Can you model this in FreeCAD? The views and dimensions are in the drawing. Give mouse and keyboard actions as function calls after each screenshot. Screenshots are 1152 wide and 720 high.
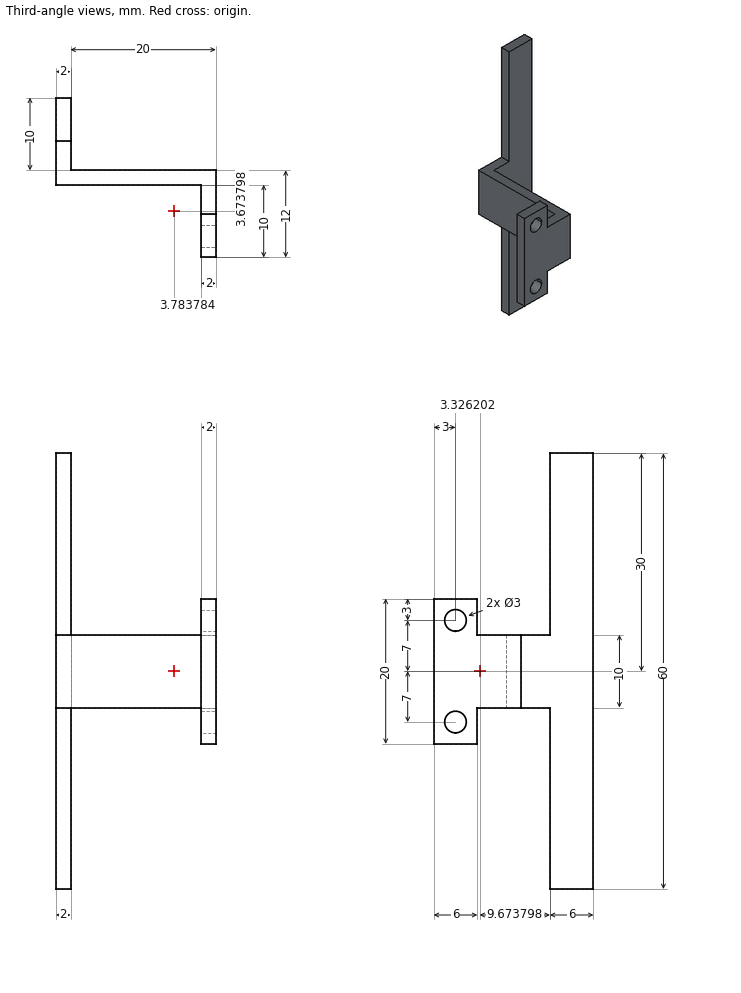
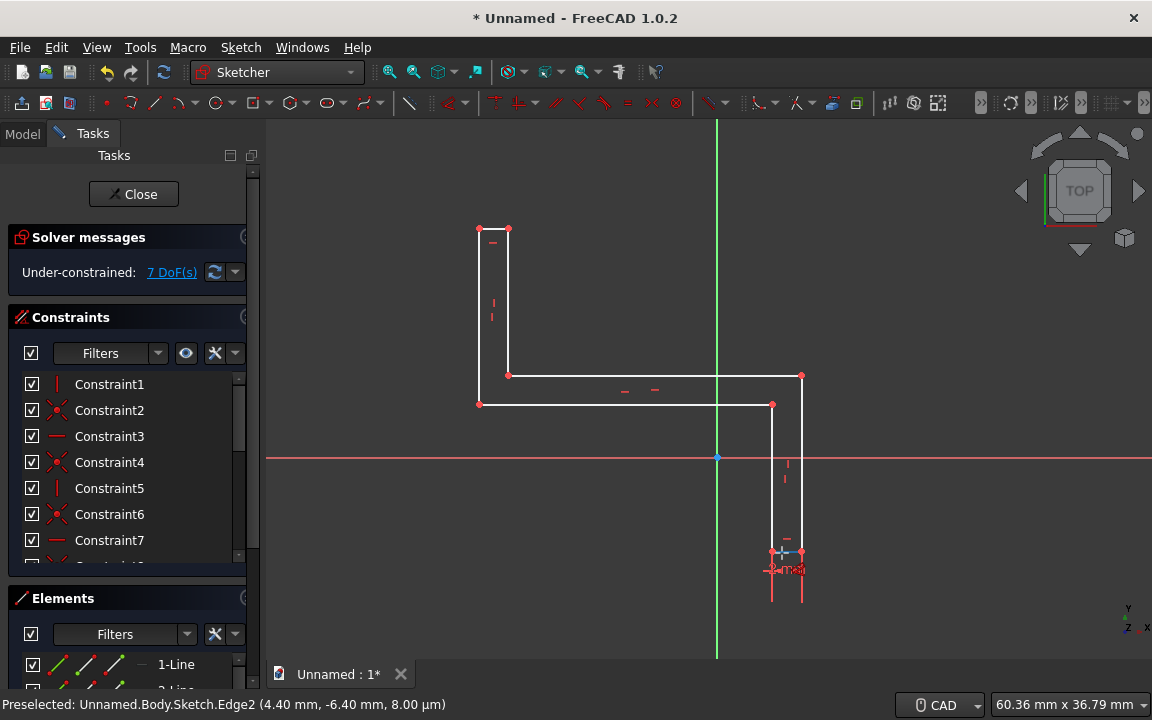
scroll(500, 229, up, 3)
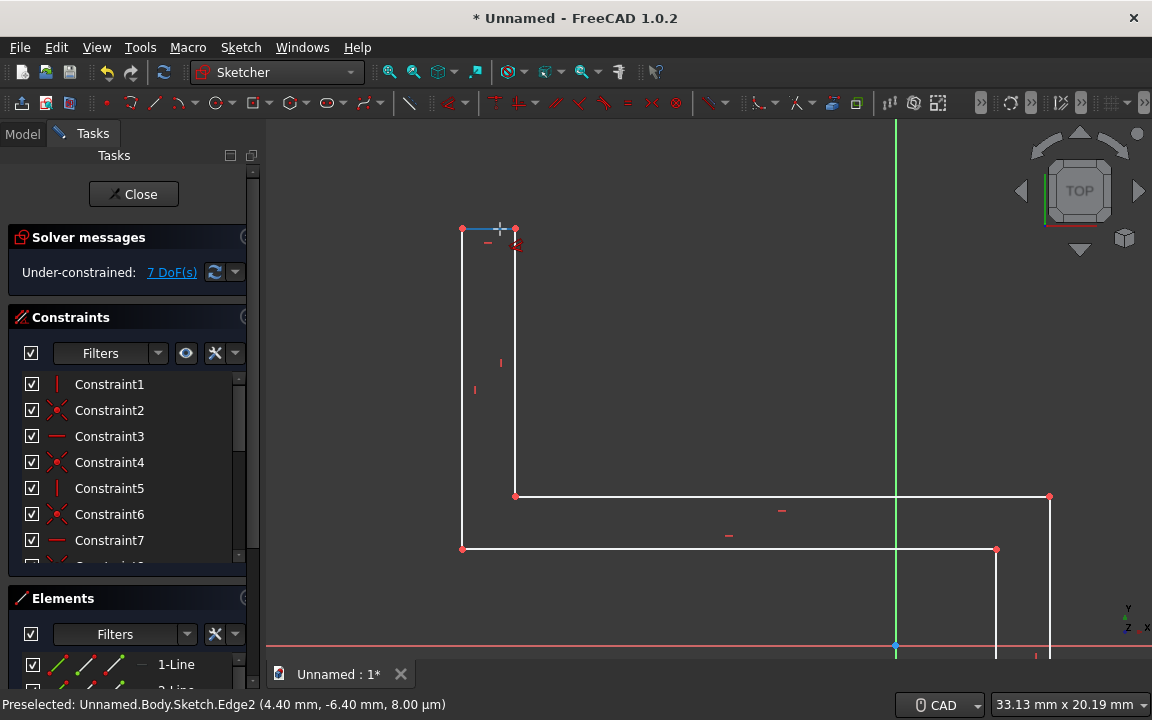
click(499, 229)
click(489, 195)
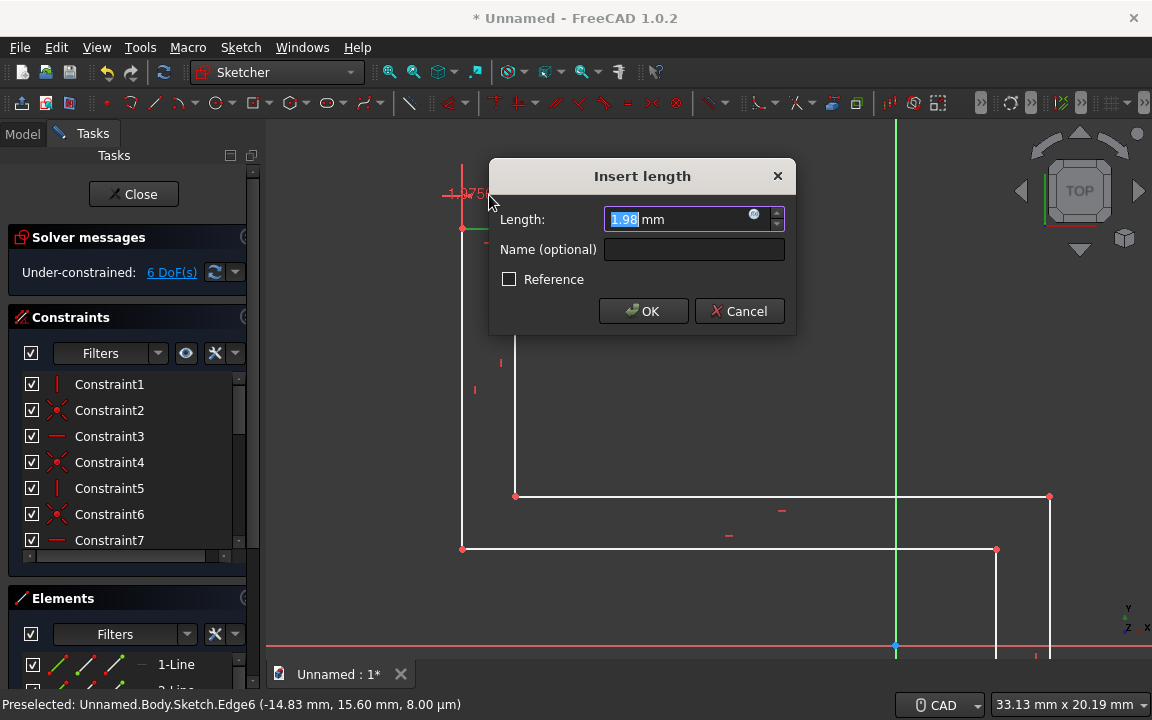
text(2)
key(Return)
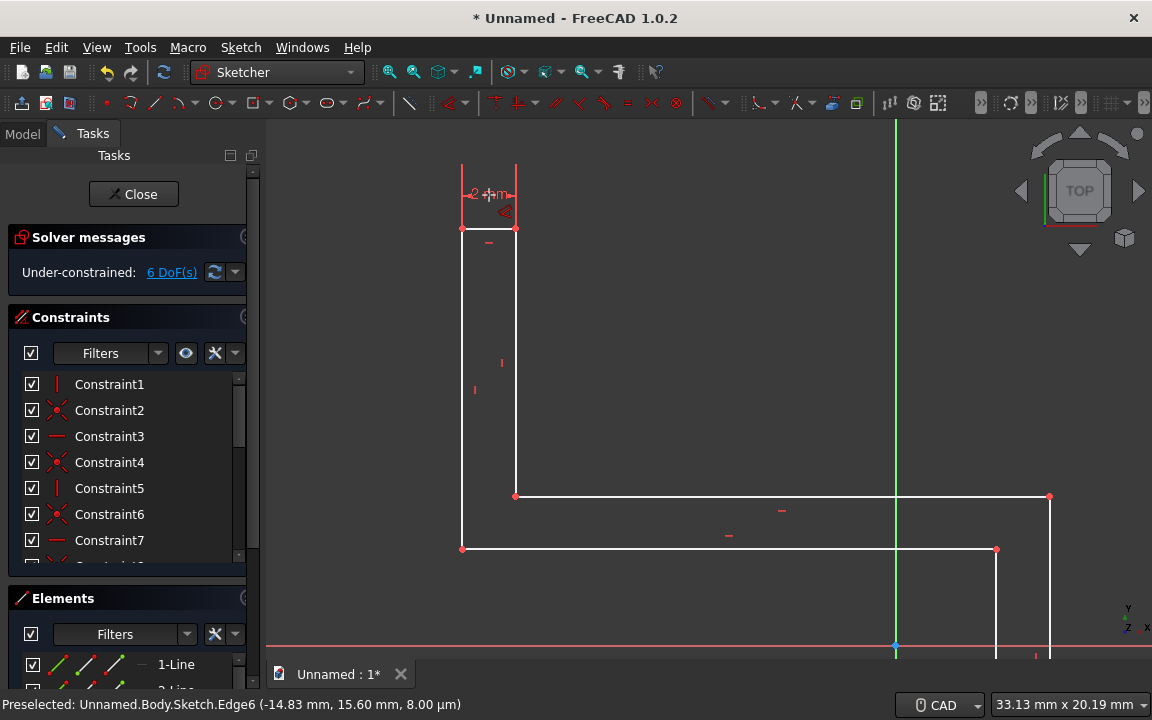
scroll(500, 229, down, 3)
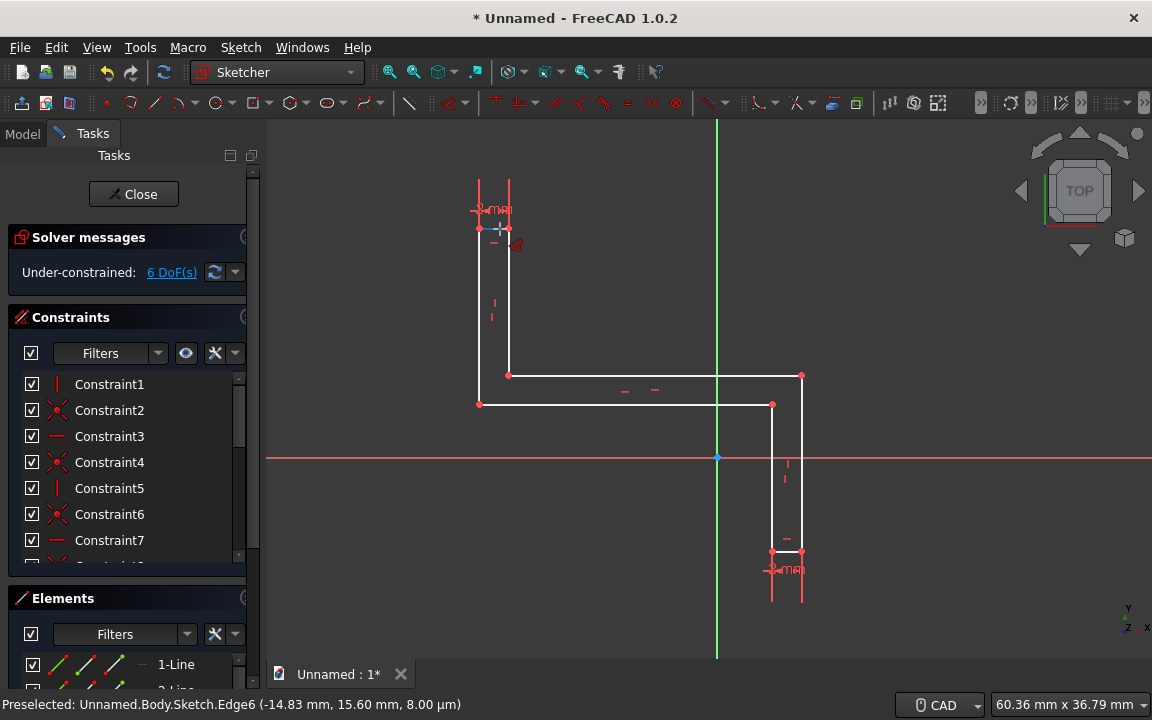
scroll(772, 449, up, 3)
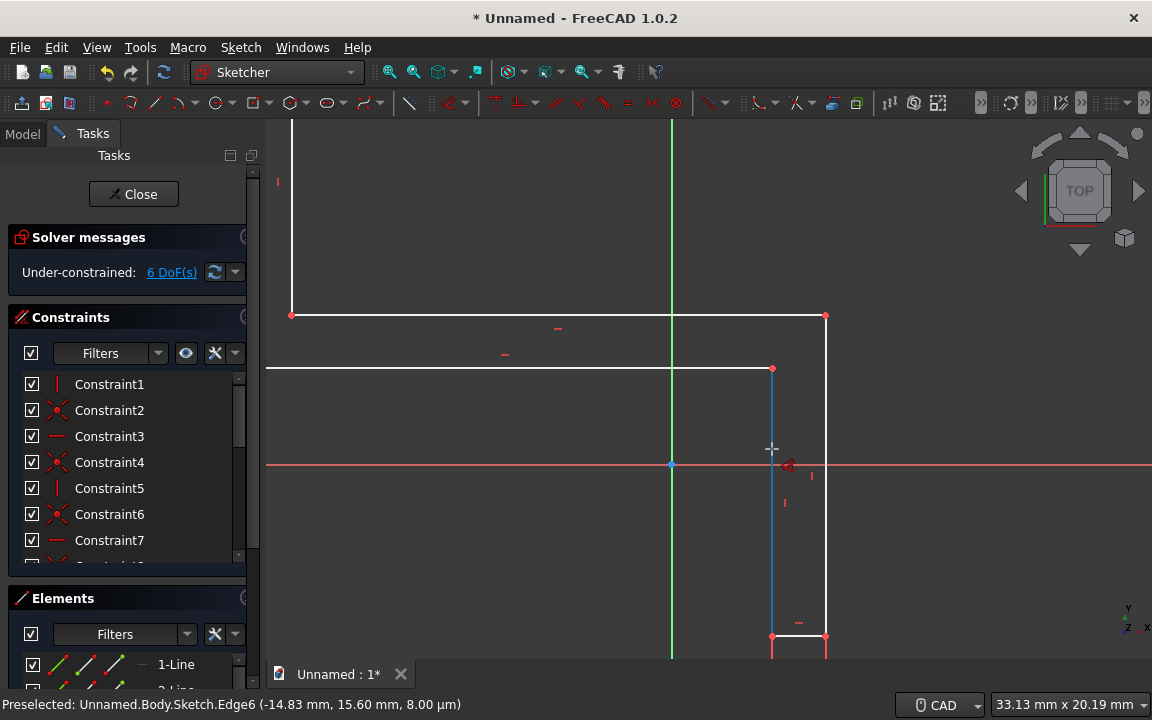
click(772, 449)
click(806, 500)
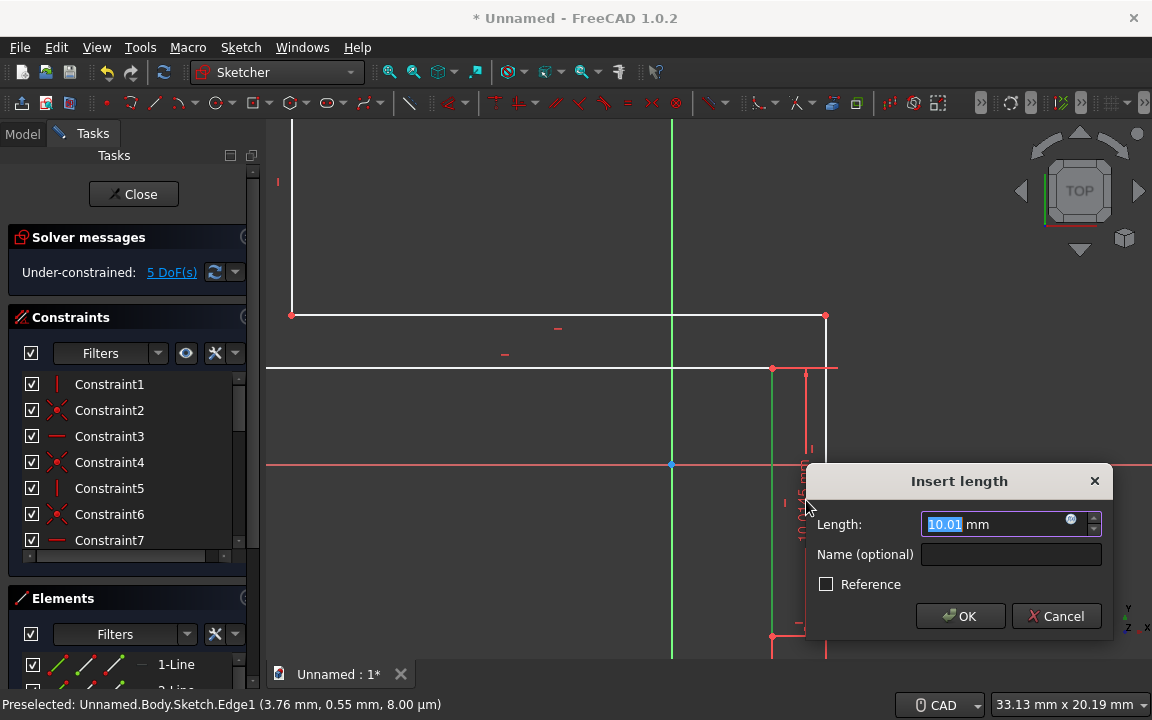
text(10)
key(Return)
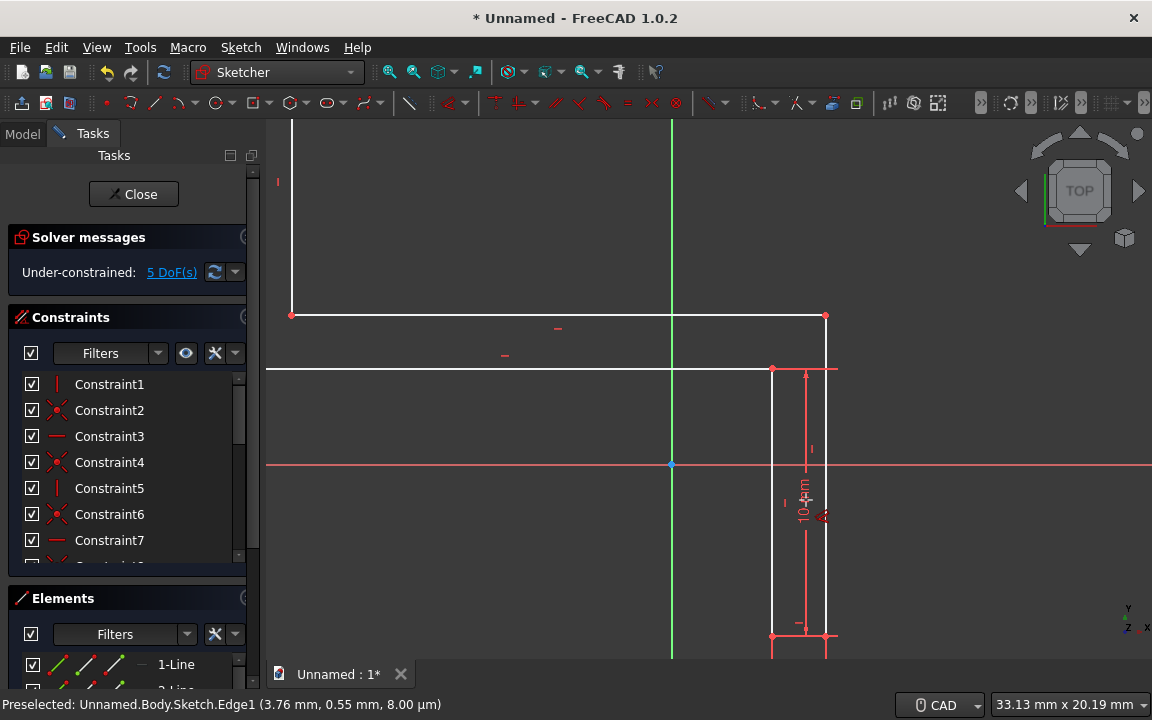
click(826, 540)
click(860, 401)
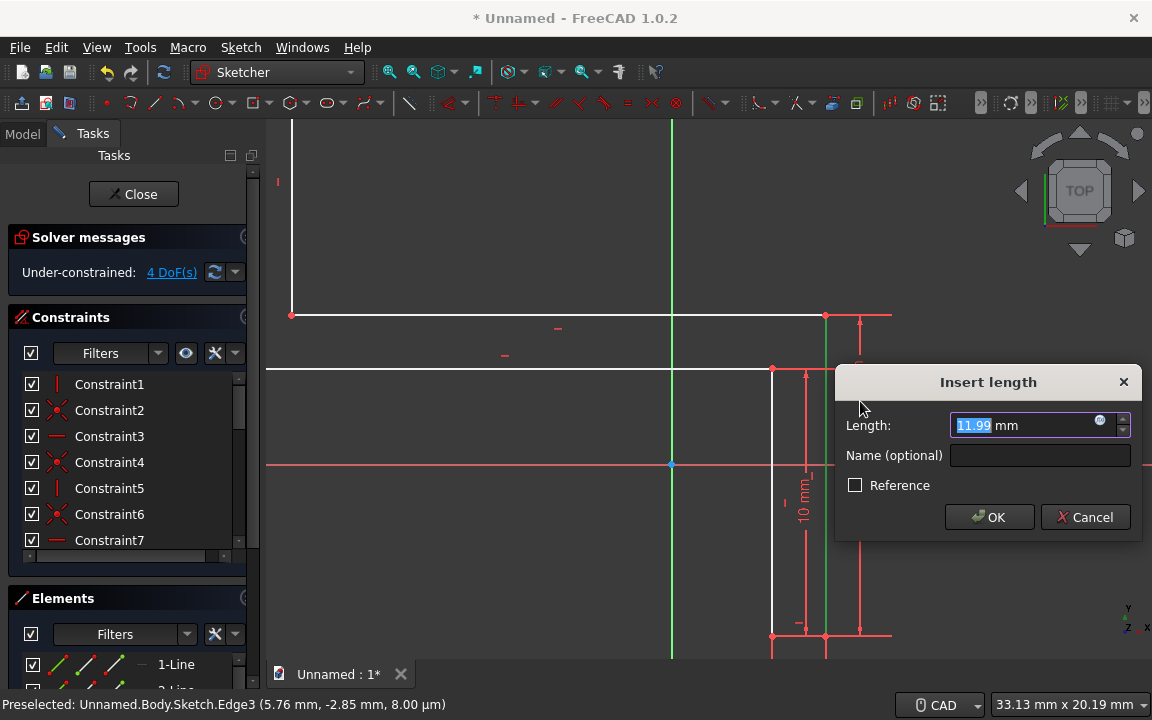
text(12)
key(Return)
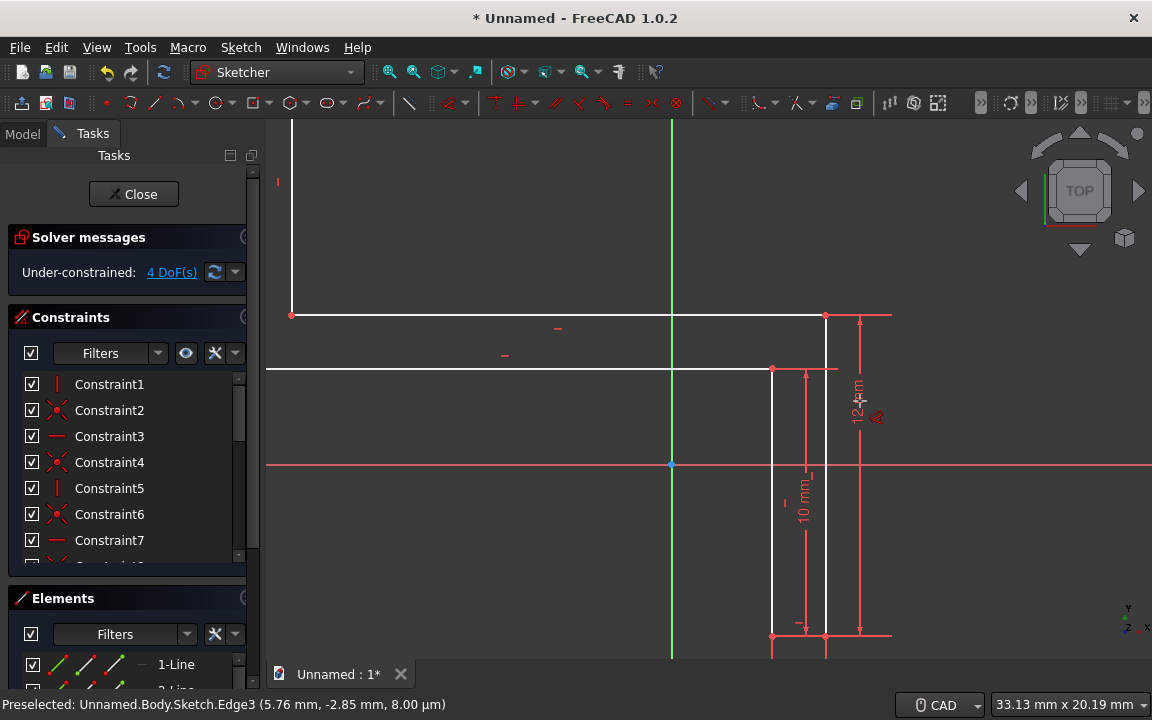
click(452, 315)
click(560, 281)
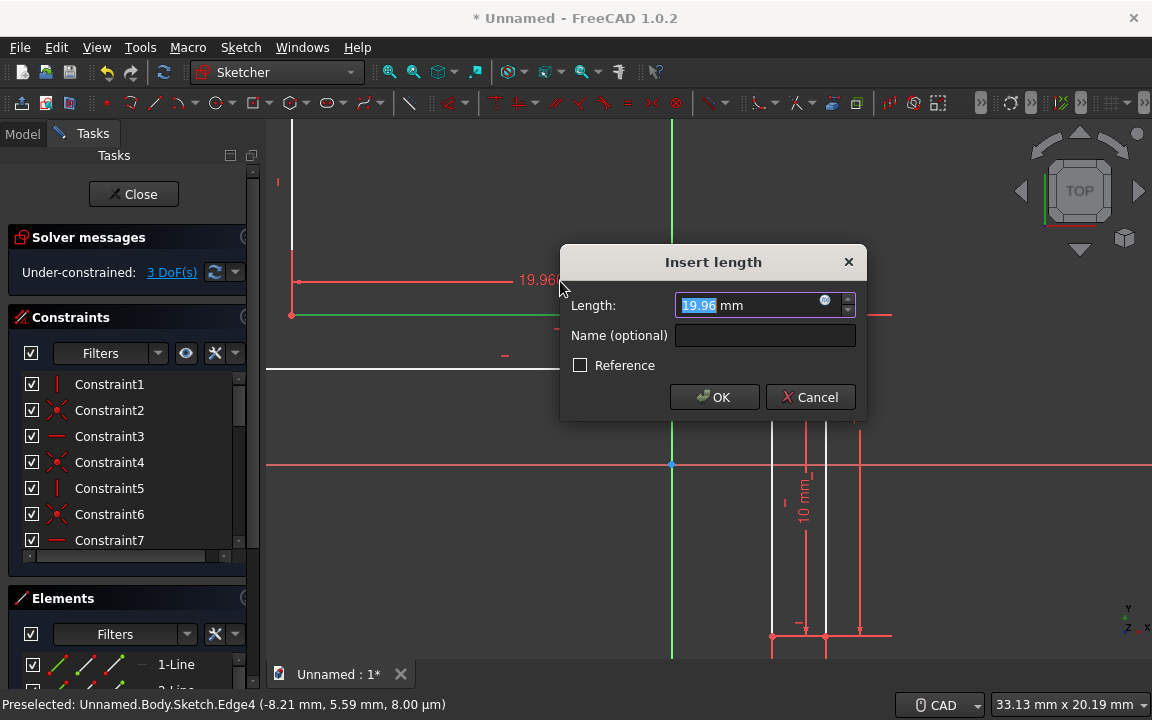
text(20)
key(Return)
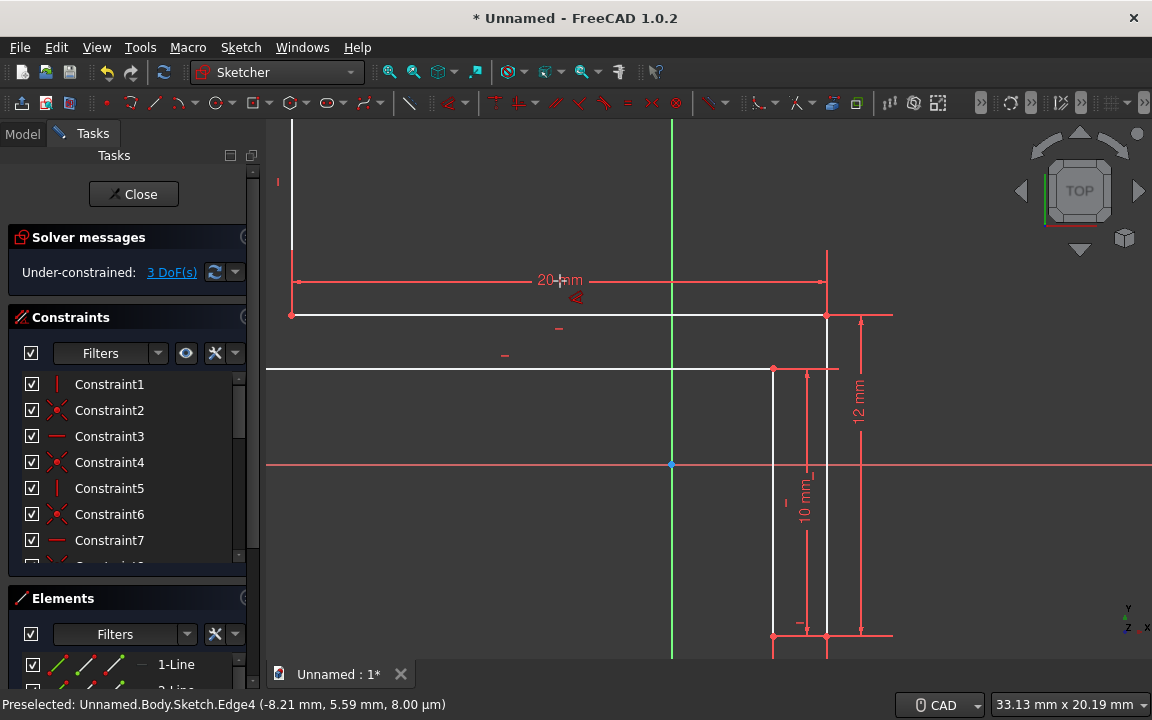
scroll(772, 449, down, 3)